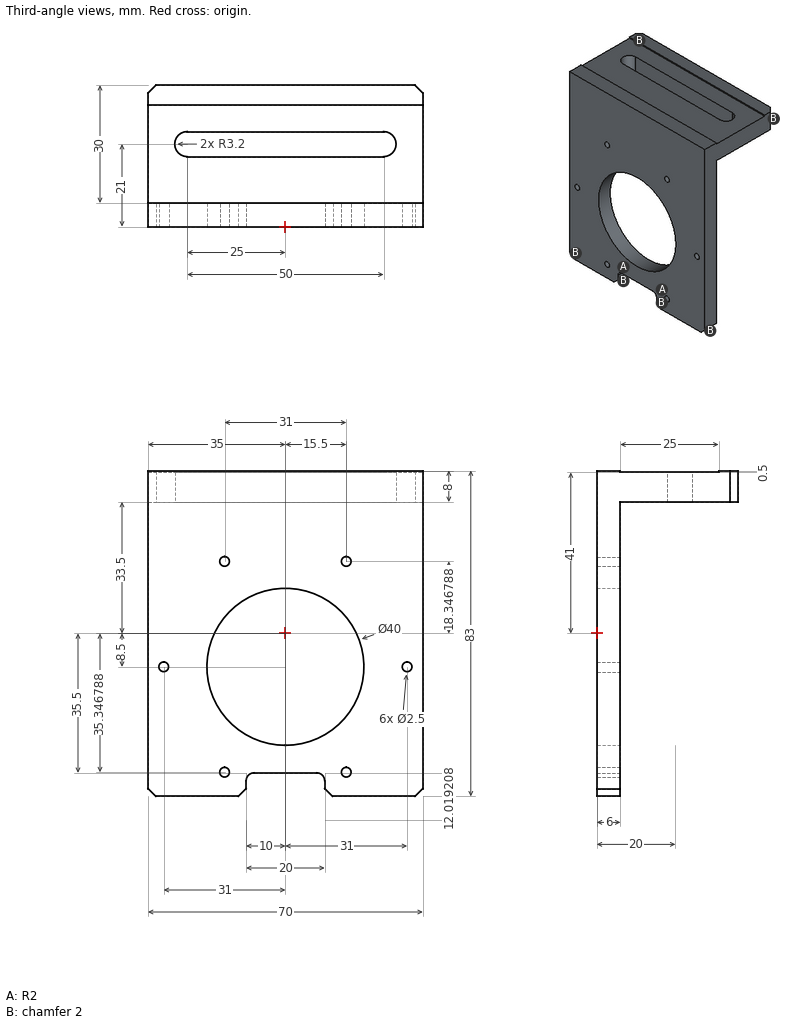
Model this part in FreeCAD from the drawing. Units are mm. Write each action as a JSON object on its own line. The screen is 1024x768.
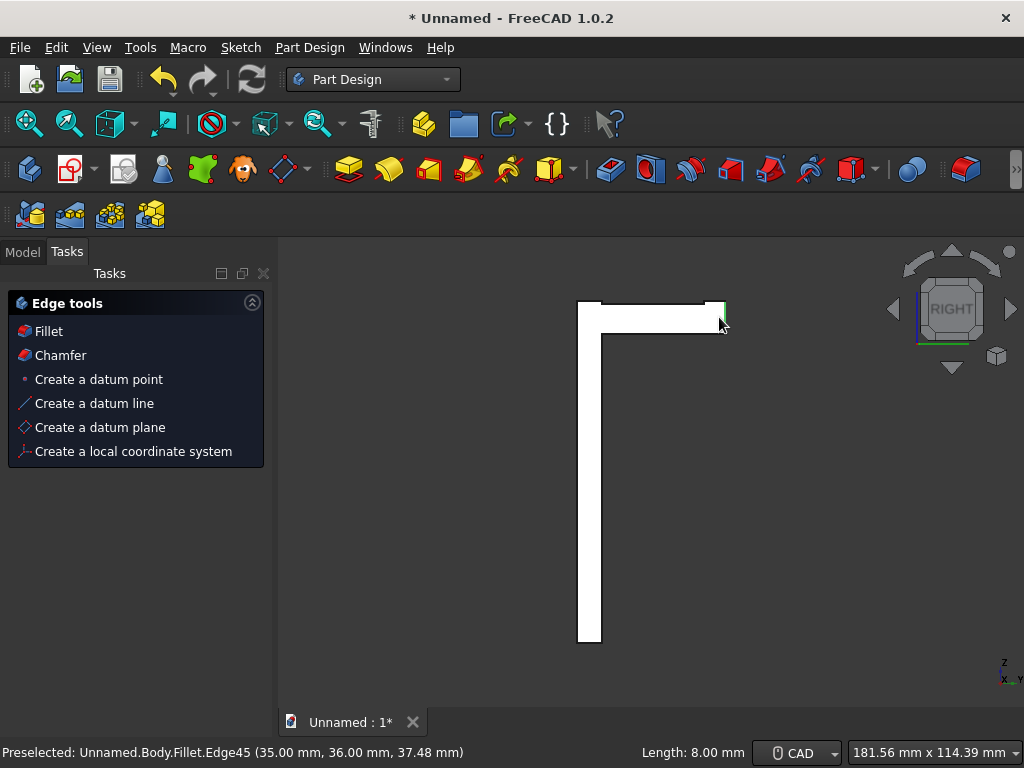
{"action": "left_click", "coordinate": [589, 642], "text": "ctrl"}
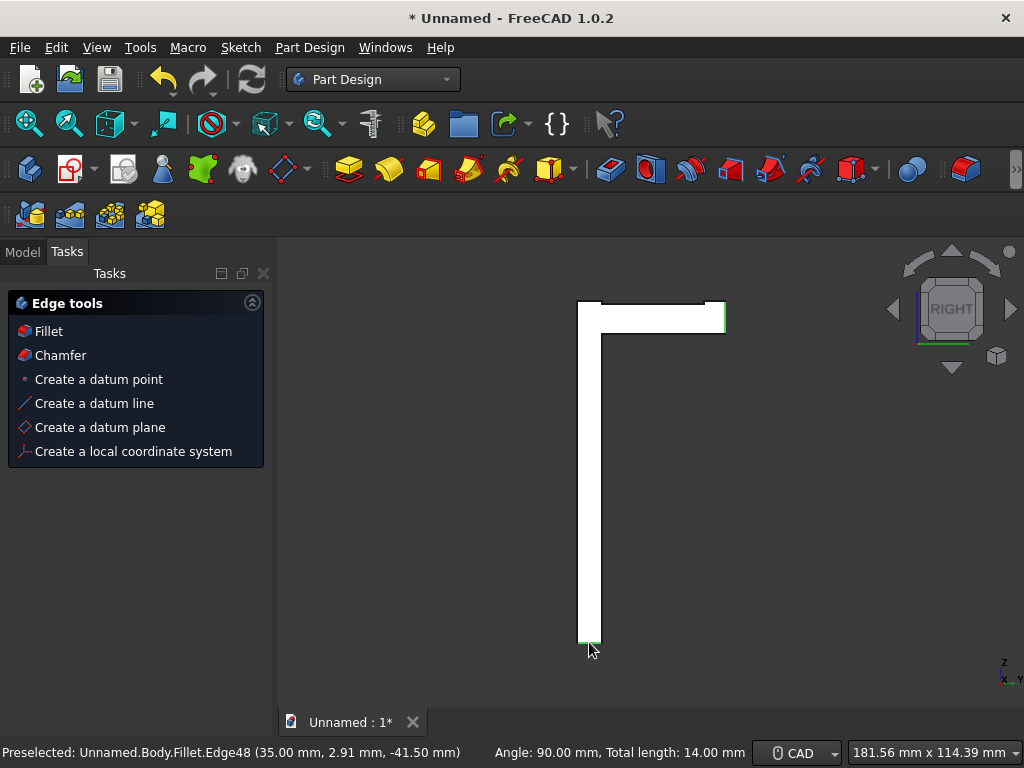
{"action": "key", "text": "5"}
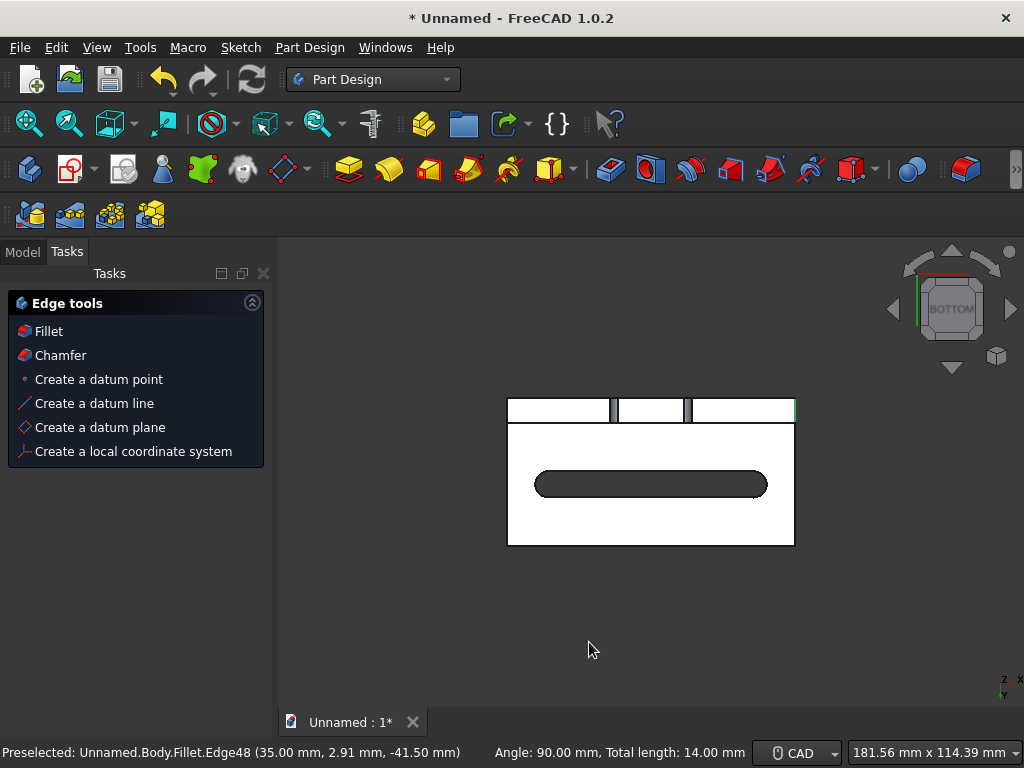
{"action": "left_click", "coordinate": [30, 124]}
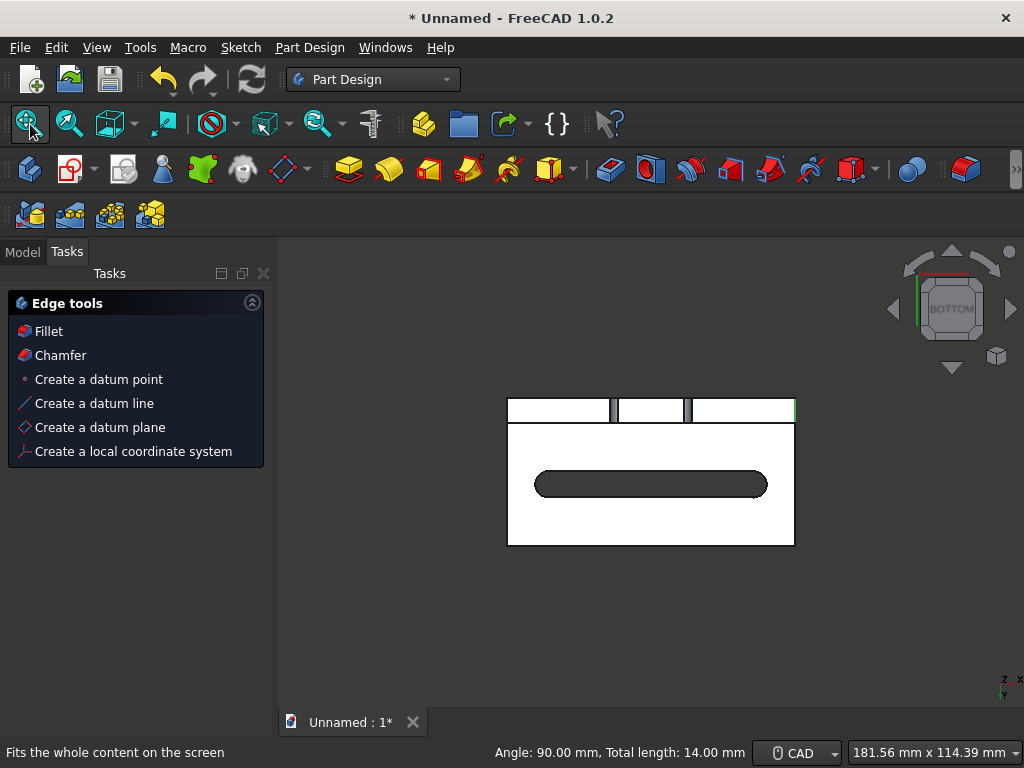
{"action": "left_click", "coordinate": [610, 409], "text": "ctrl"}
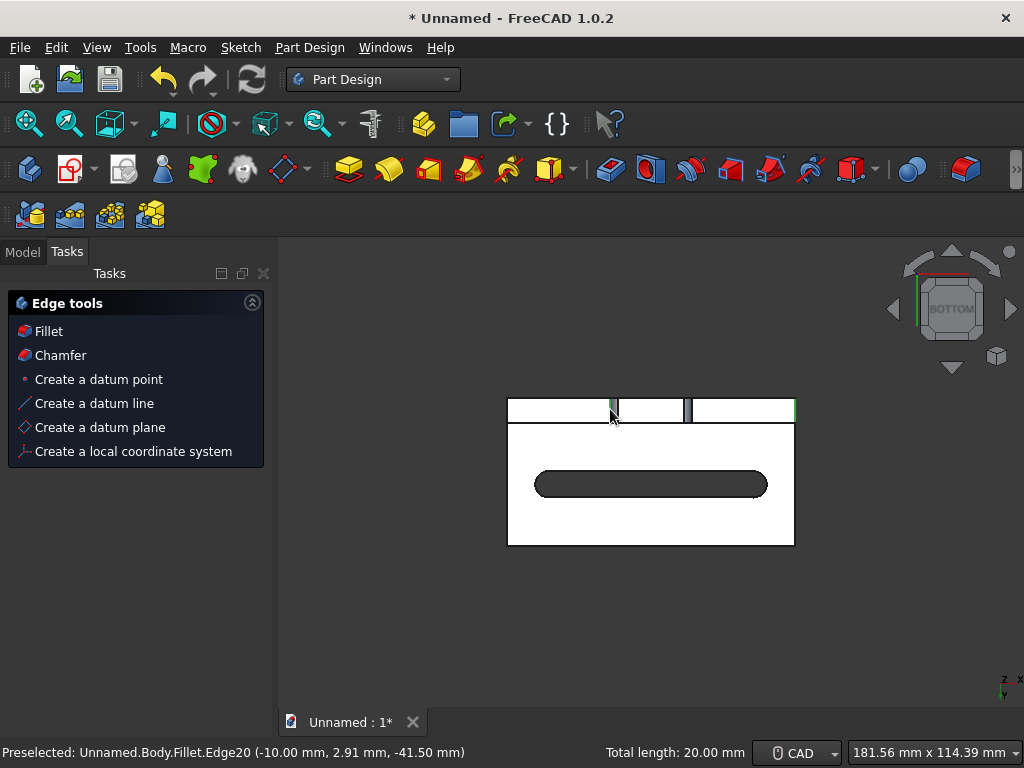
{"action": "left_click", "coordinate": [692, 409], "text": "ctrl"}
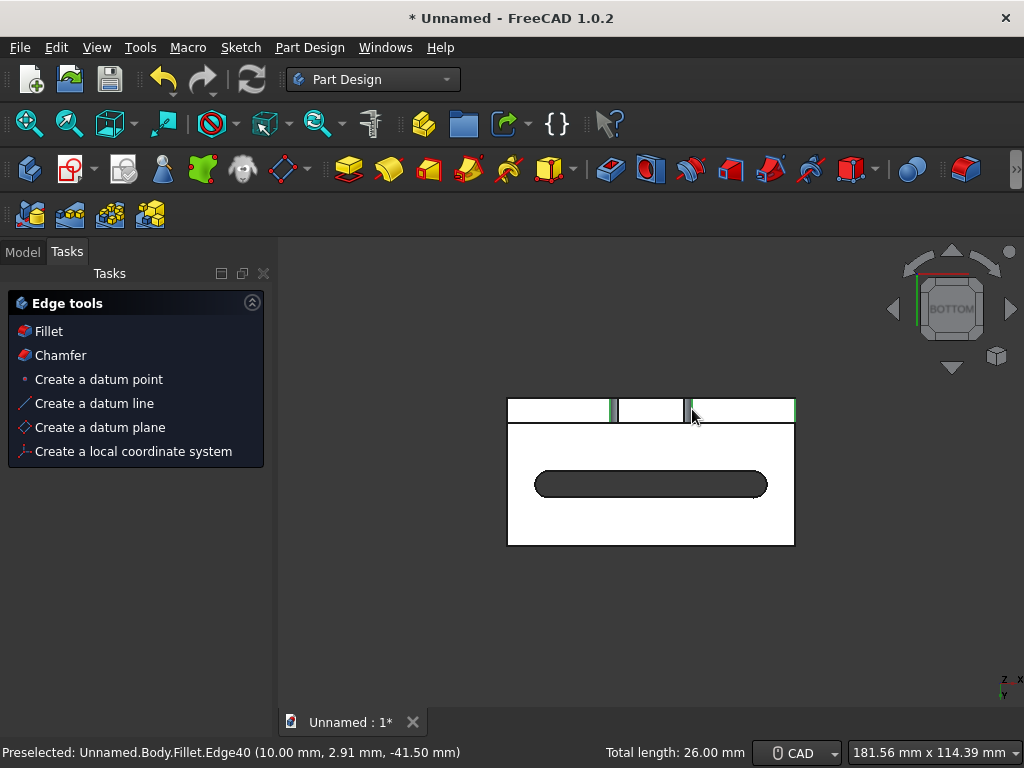
{"action": "left_click", "coordinate": [507, 409], "text": "ctrl"}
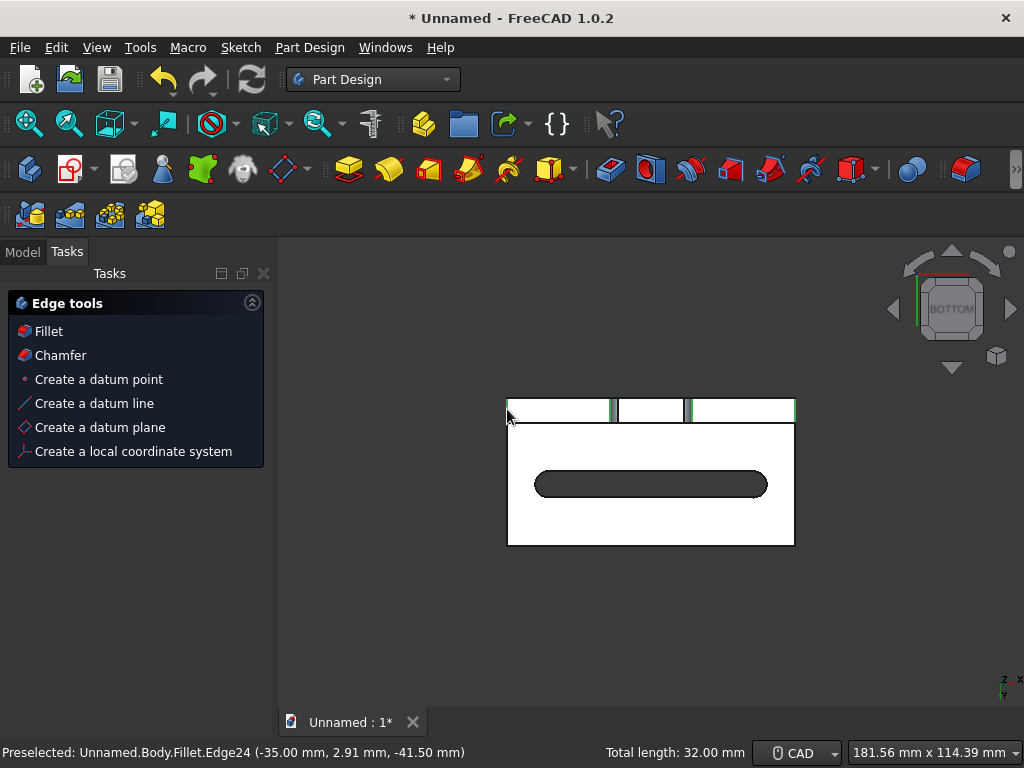
{"action": "key", "text": "4"}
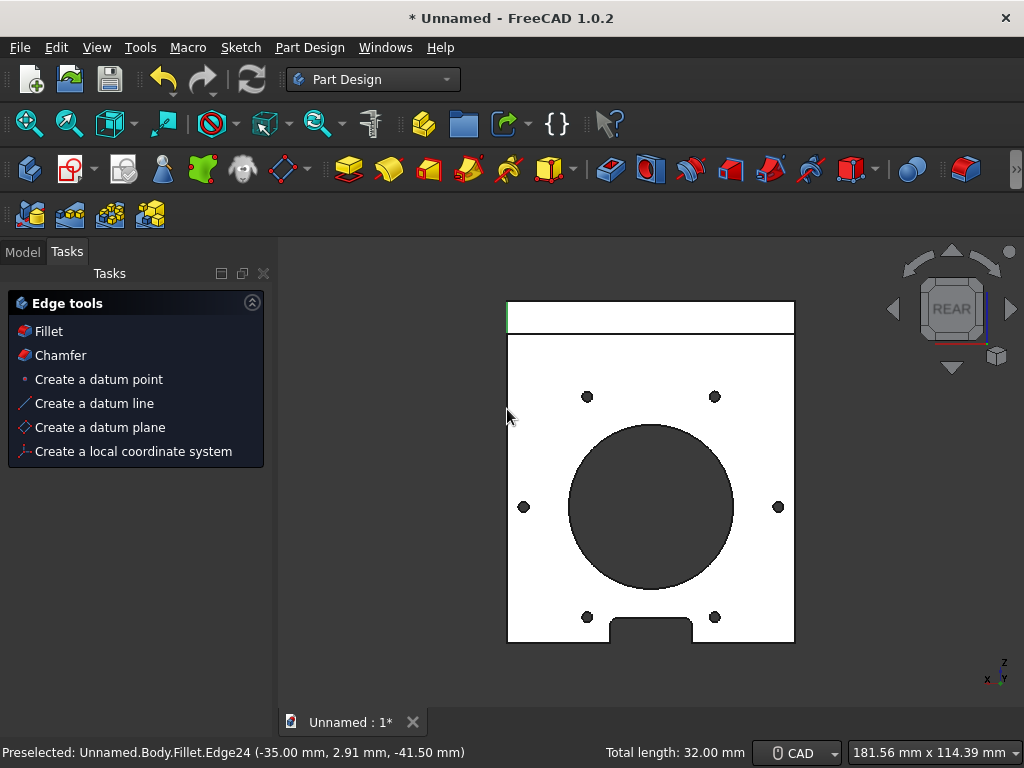
{"action": "left_click", "coordinate": [795, 317], "text": "ctrl"}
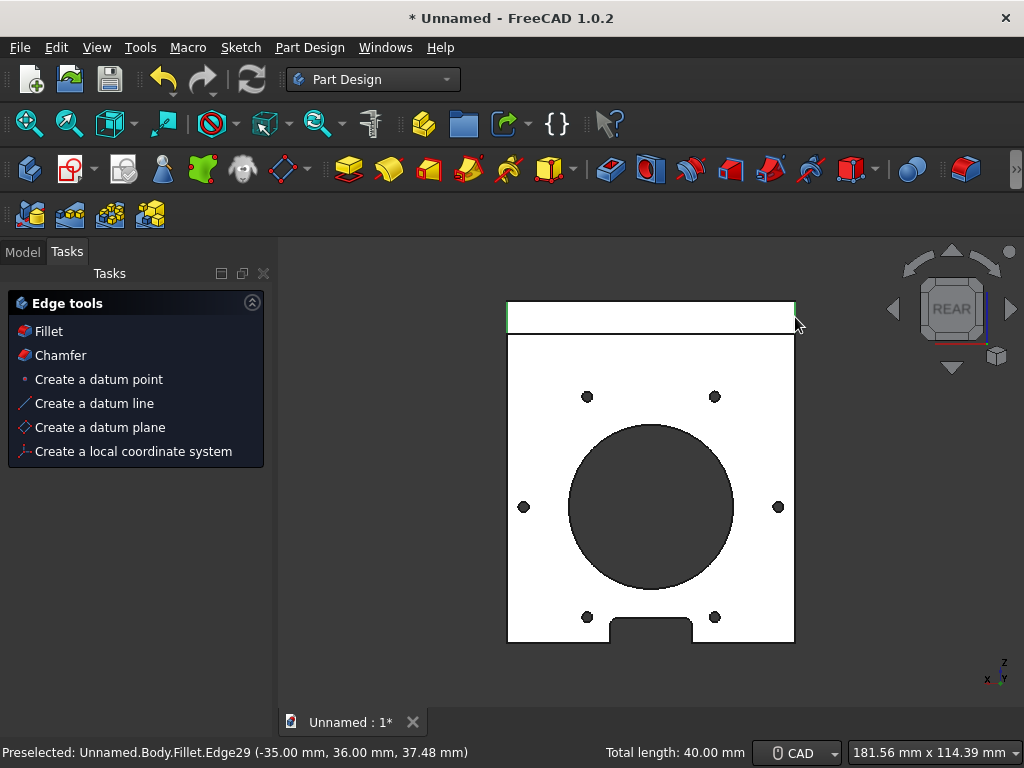
{"action": "left_click", "coordinate": [136, 355]}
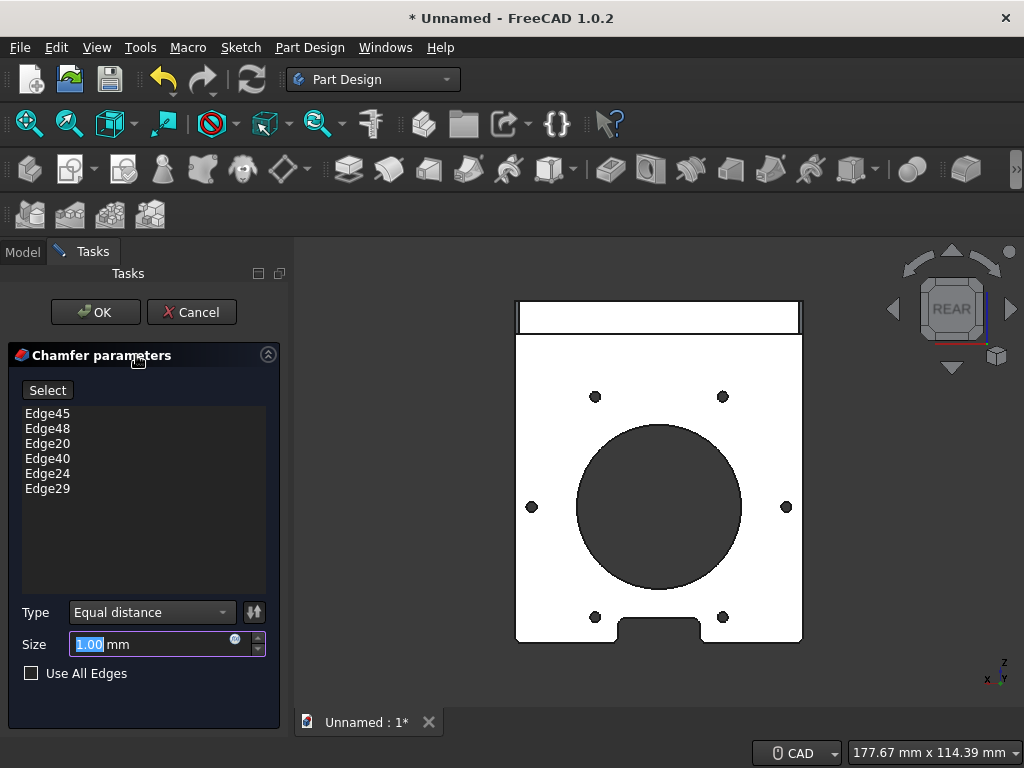
{"action": "type", "text": "2"}
{"action": "key", "text": "Tab"}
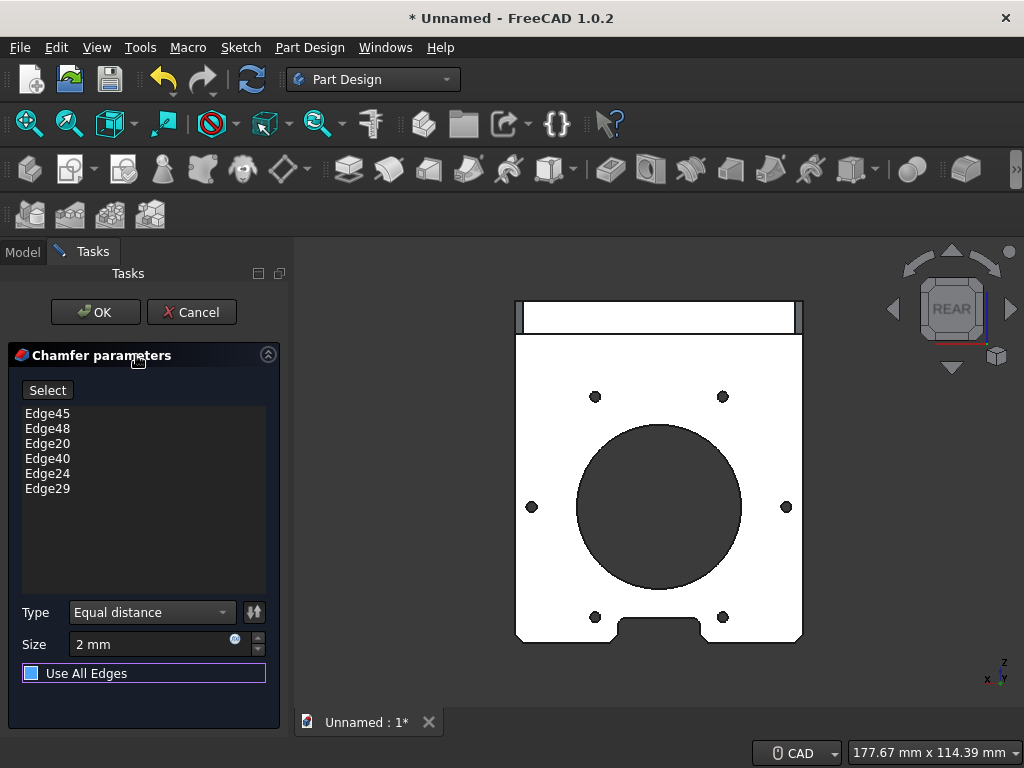
{"action": "left_click", "coordinate": [96, 312]}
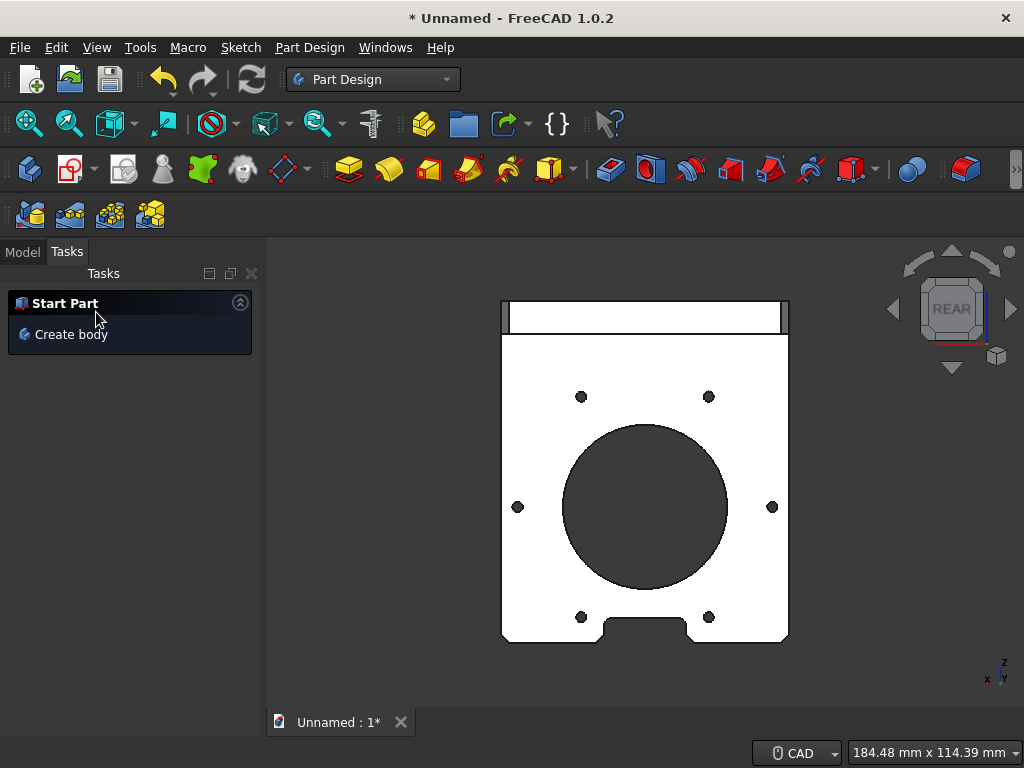
{"action": "key", "text": "0"}